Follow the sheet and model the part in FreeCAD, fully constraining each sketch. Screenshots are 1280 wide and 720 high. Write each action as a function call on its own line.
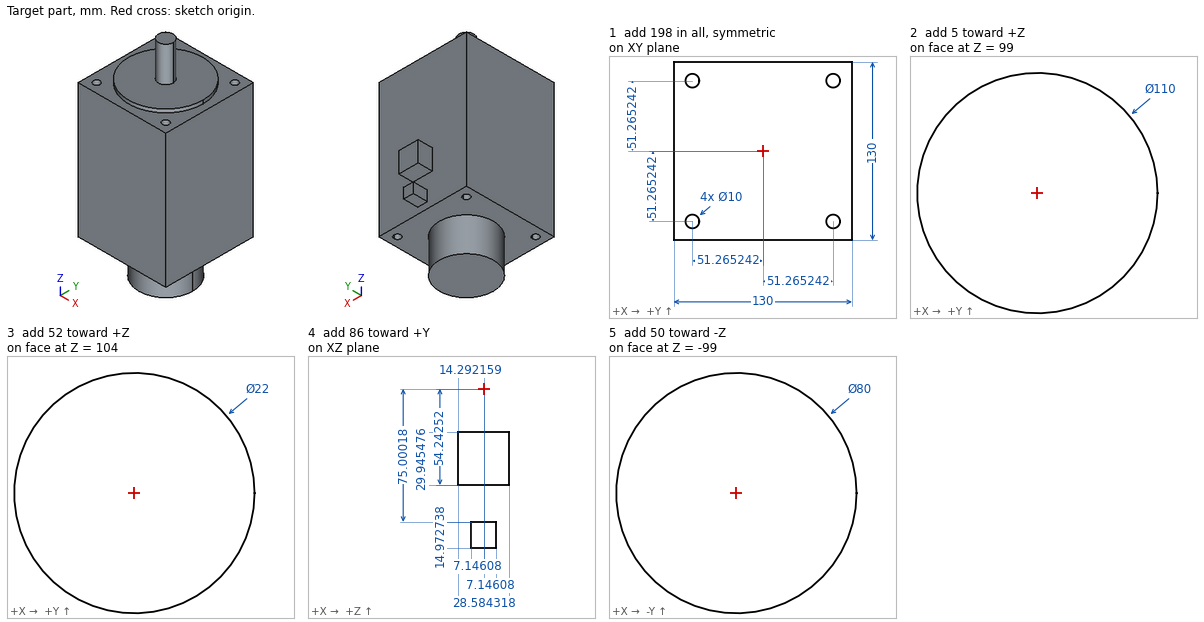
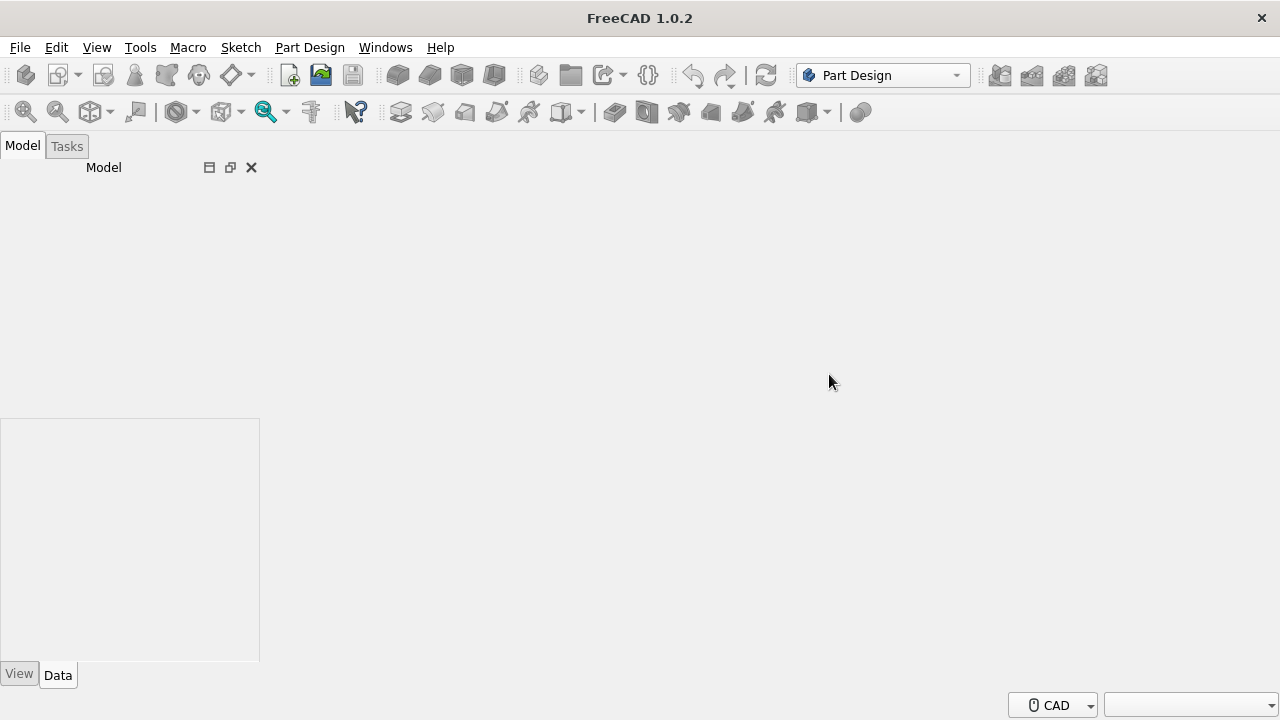
key(ctrl+n)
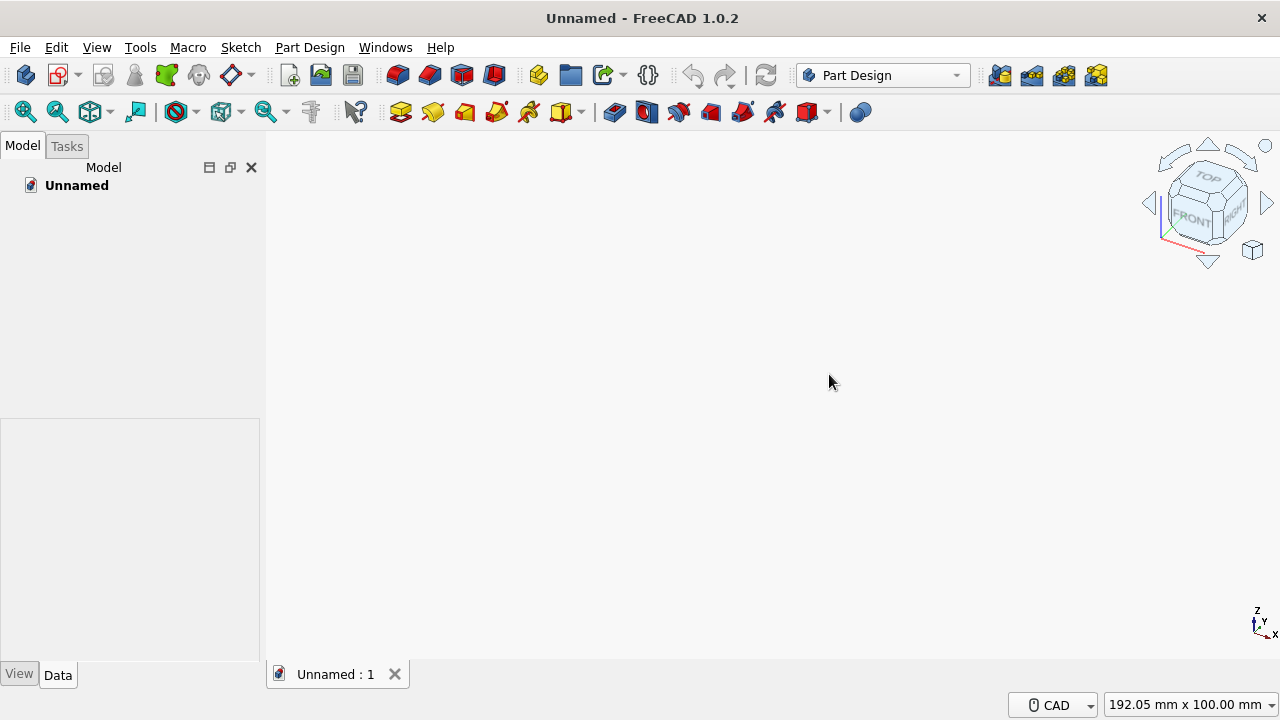
click(58, 76)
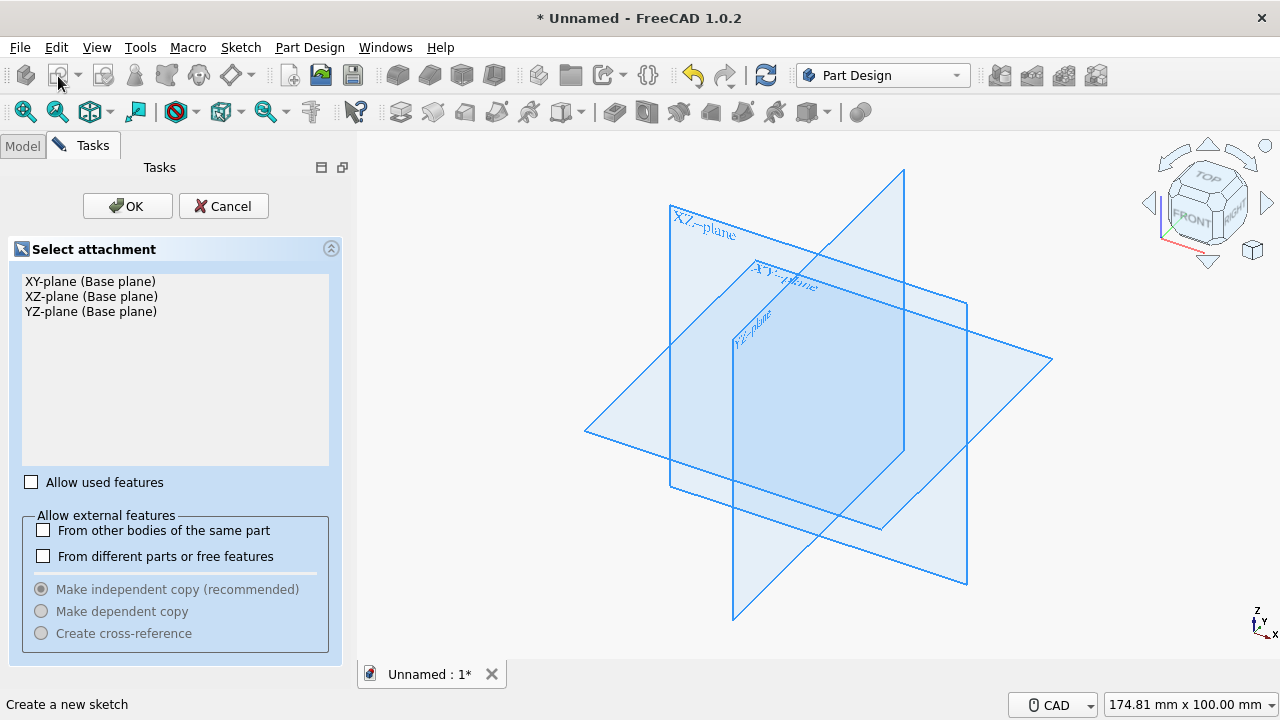
click(82, 282)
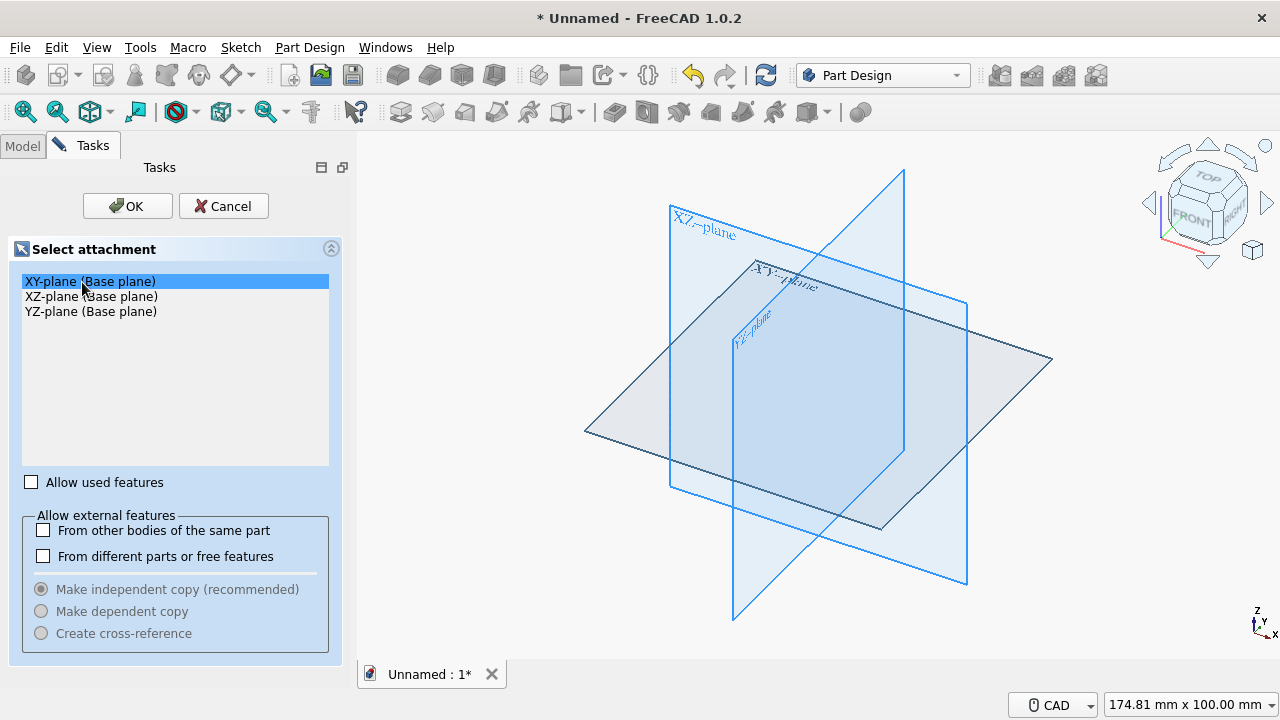
click(128, 206)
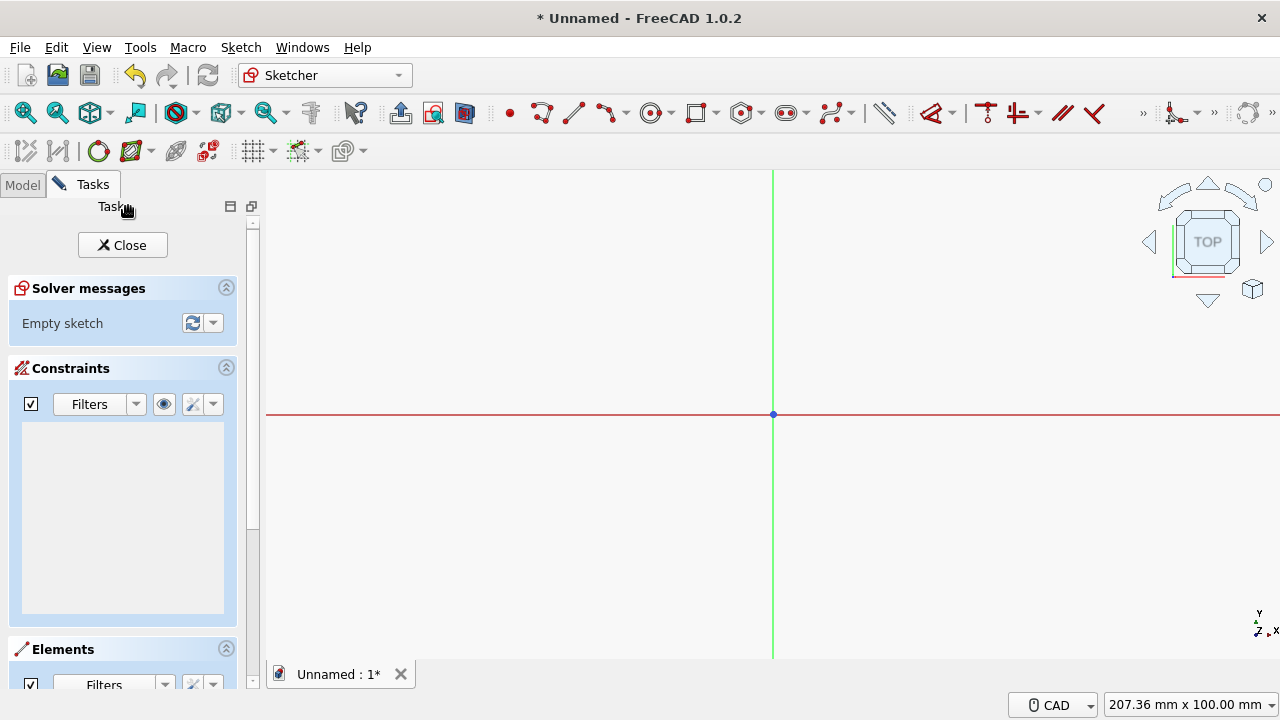
scroll(649, 414, down, 4)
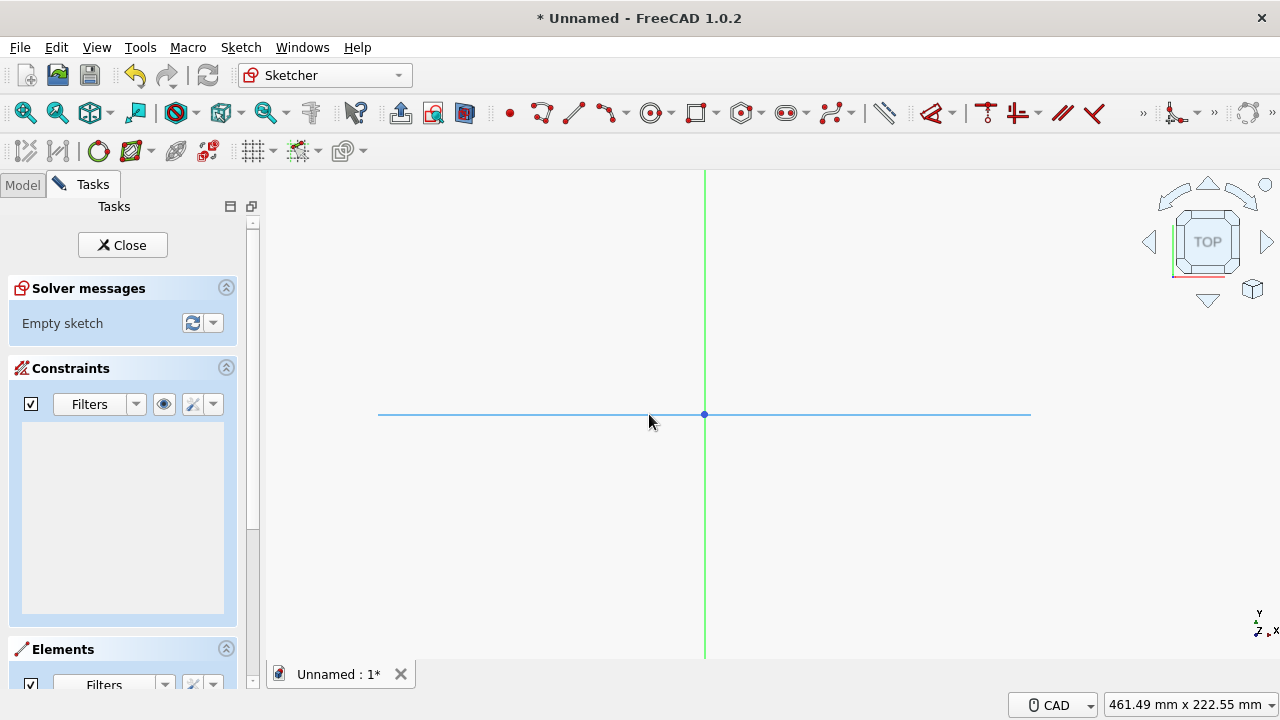
key(g)
key(v)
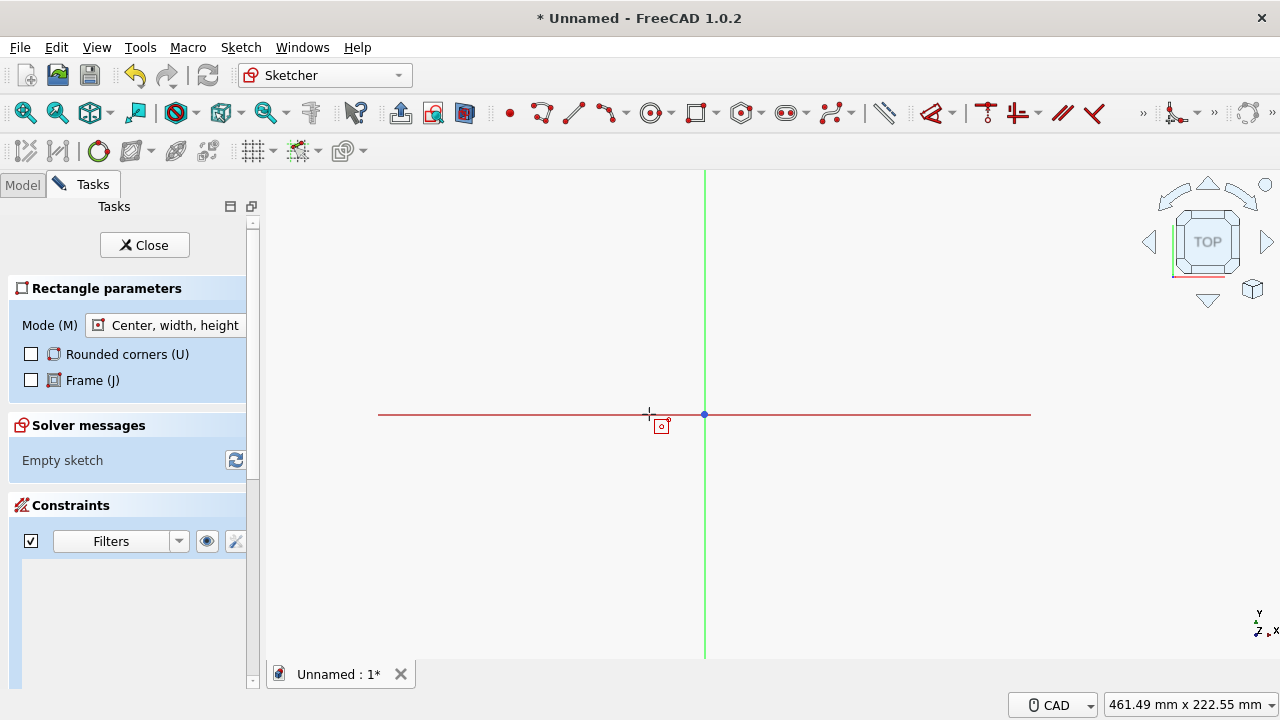
click(705, 414)
click(848, 272)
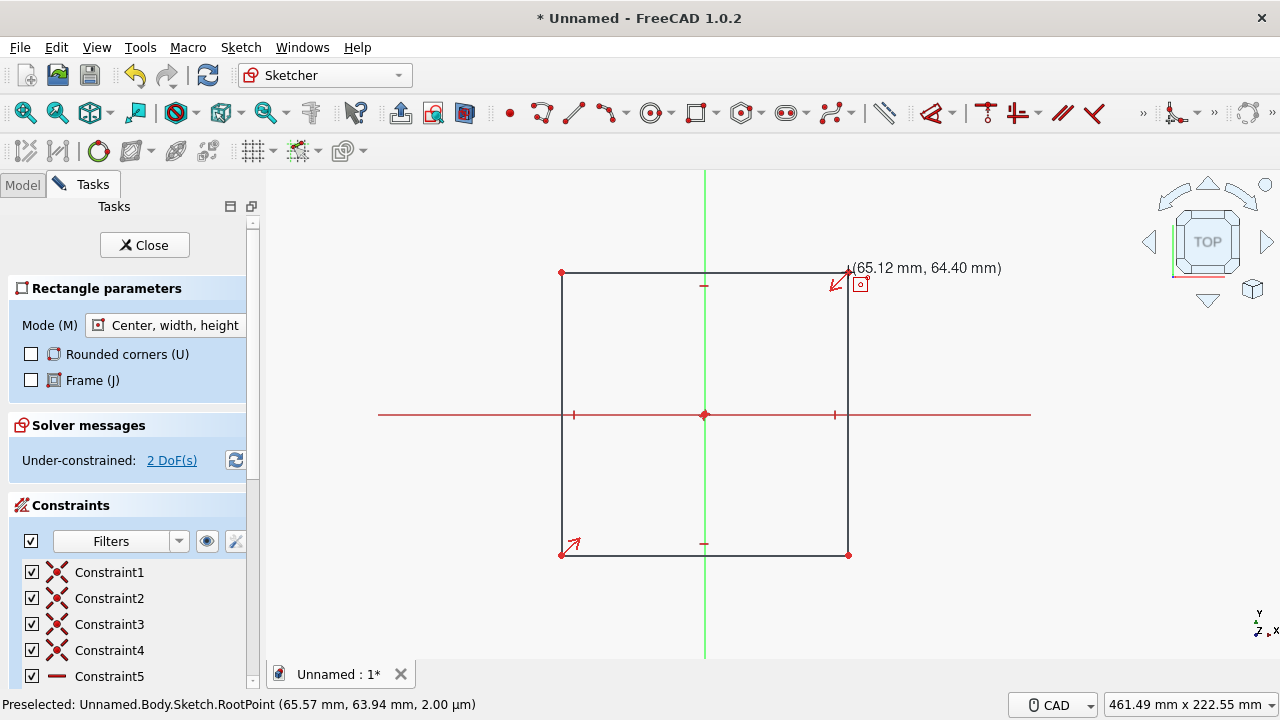
click(652, 114)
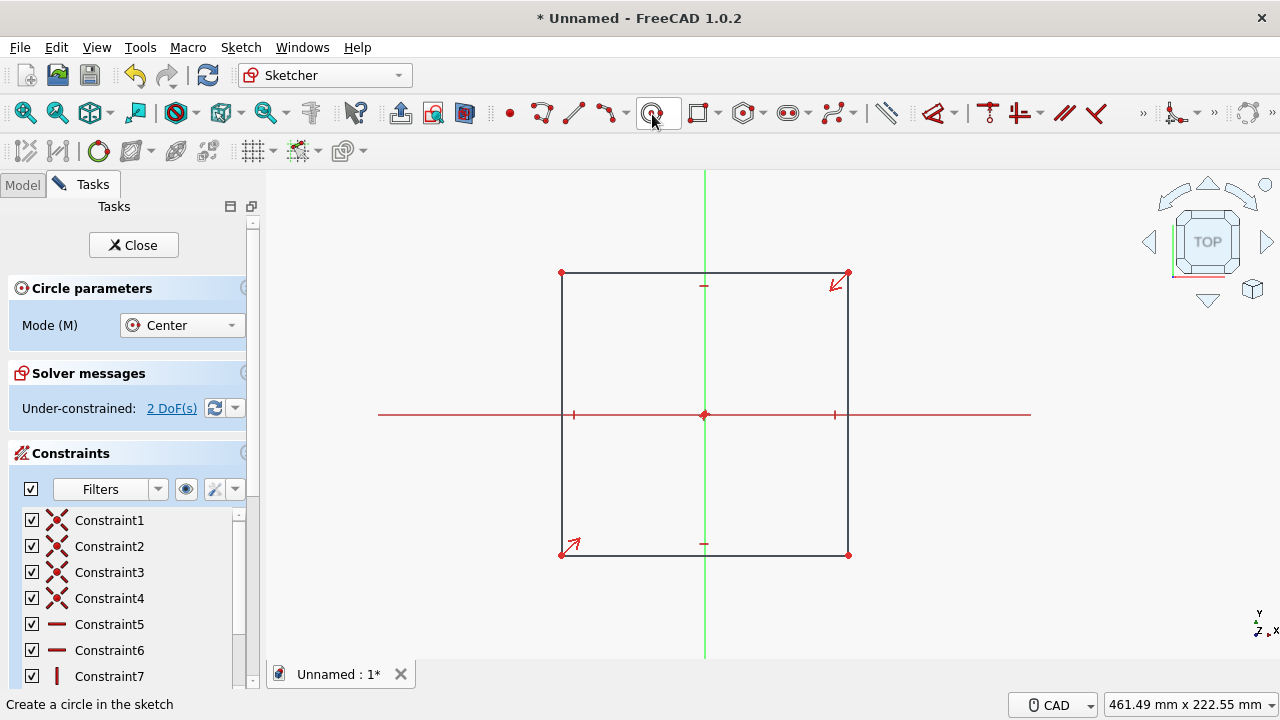
scroll(592, 527, up, 4)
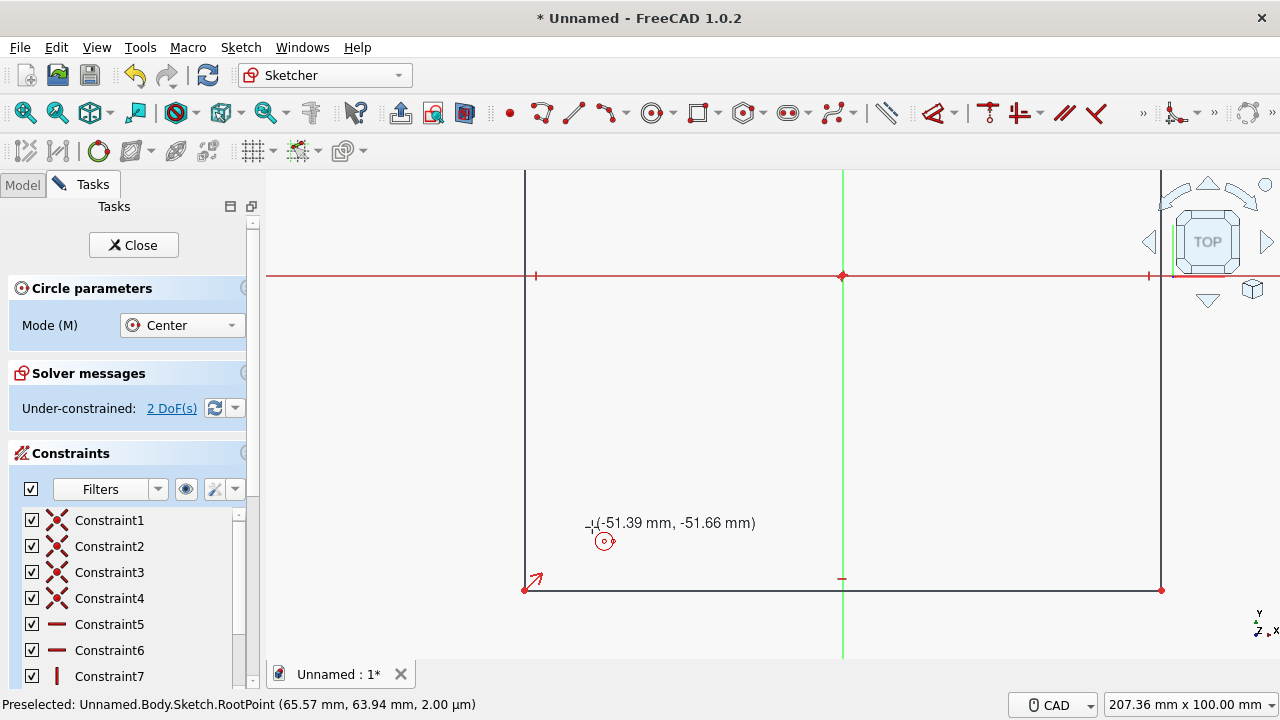
click(592, 526)
click(610, 509)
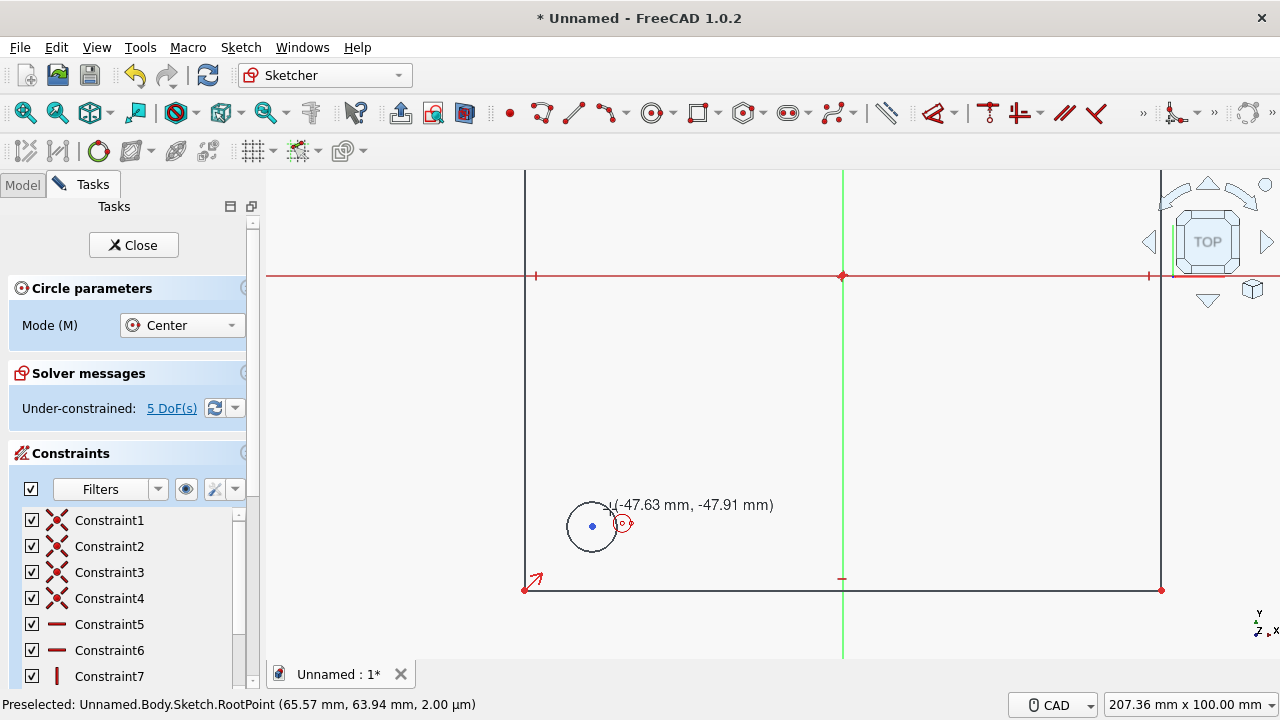
click(1094, 526)
click(1111, 509)